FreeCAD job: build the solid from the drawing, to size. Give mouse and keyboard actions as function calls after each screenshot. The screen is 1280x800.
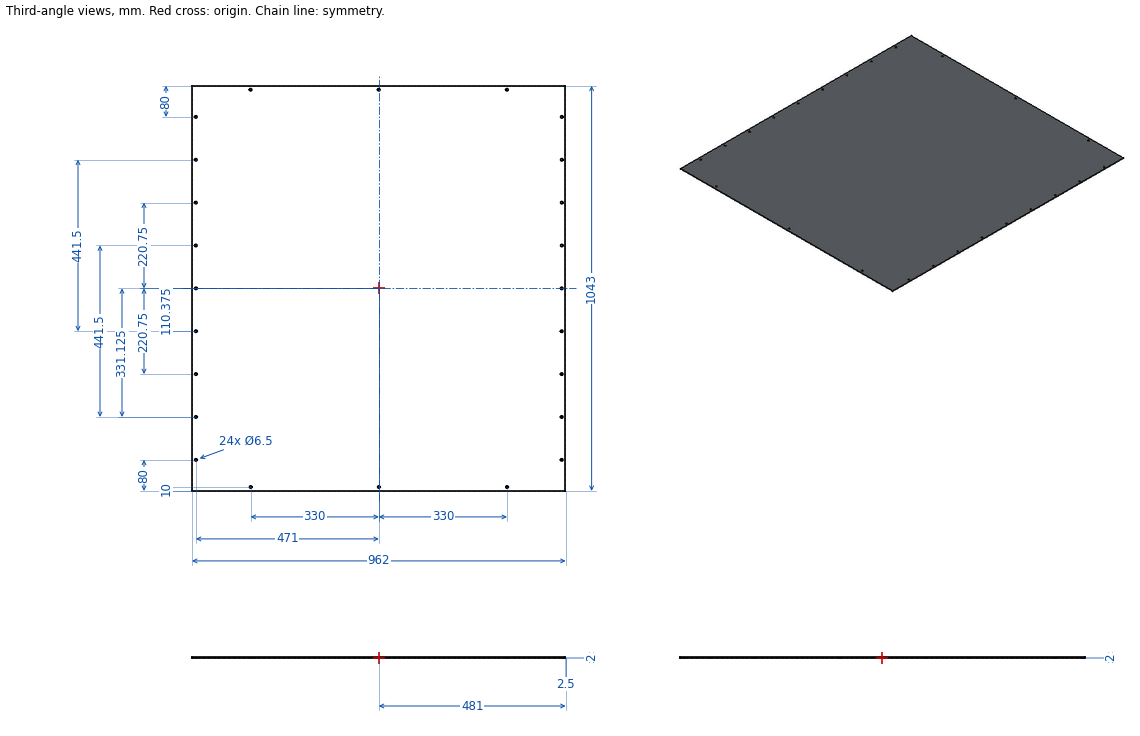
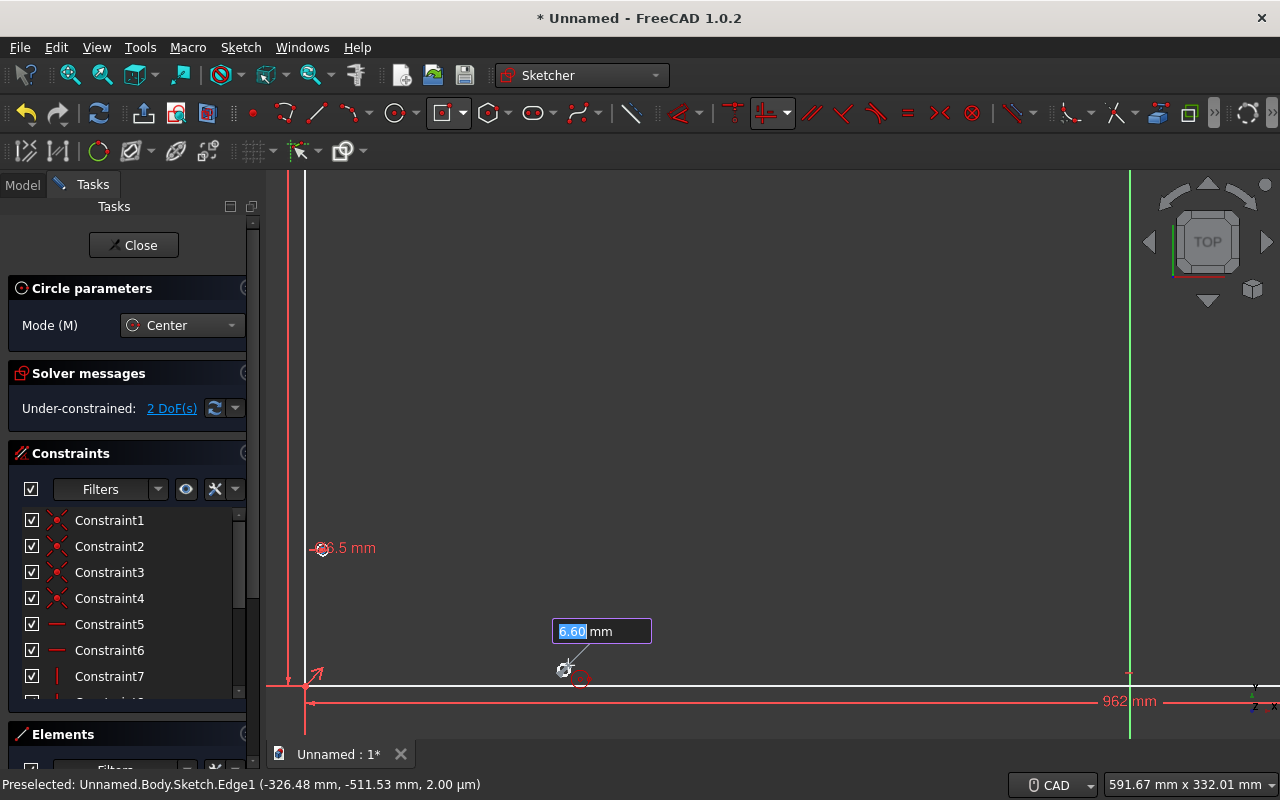
text(6.5)
key(Return)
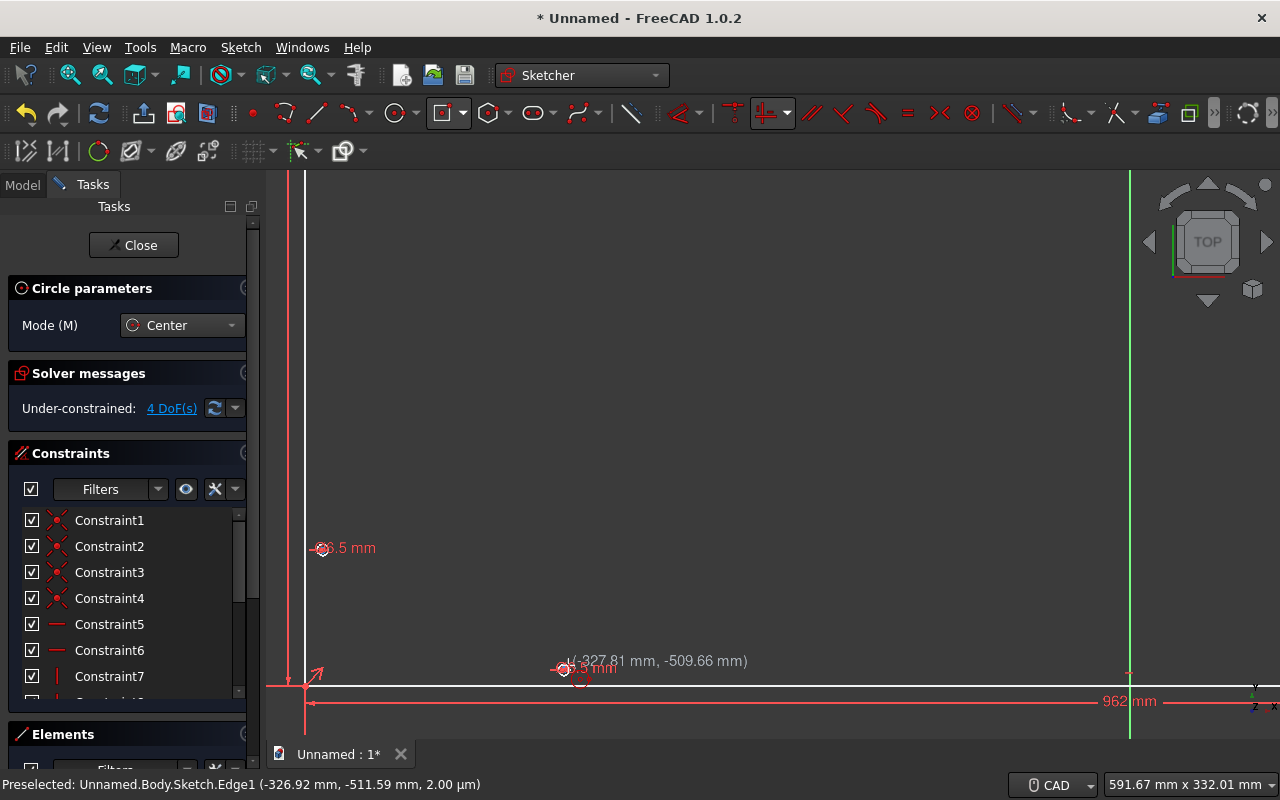
scroll(323, 360, up, 8)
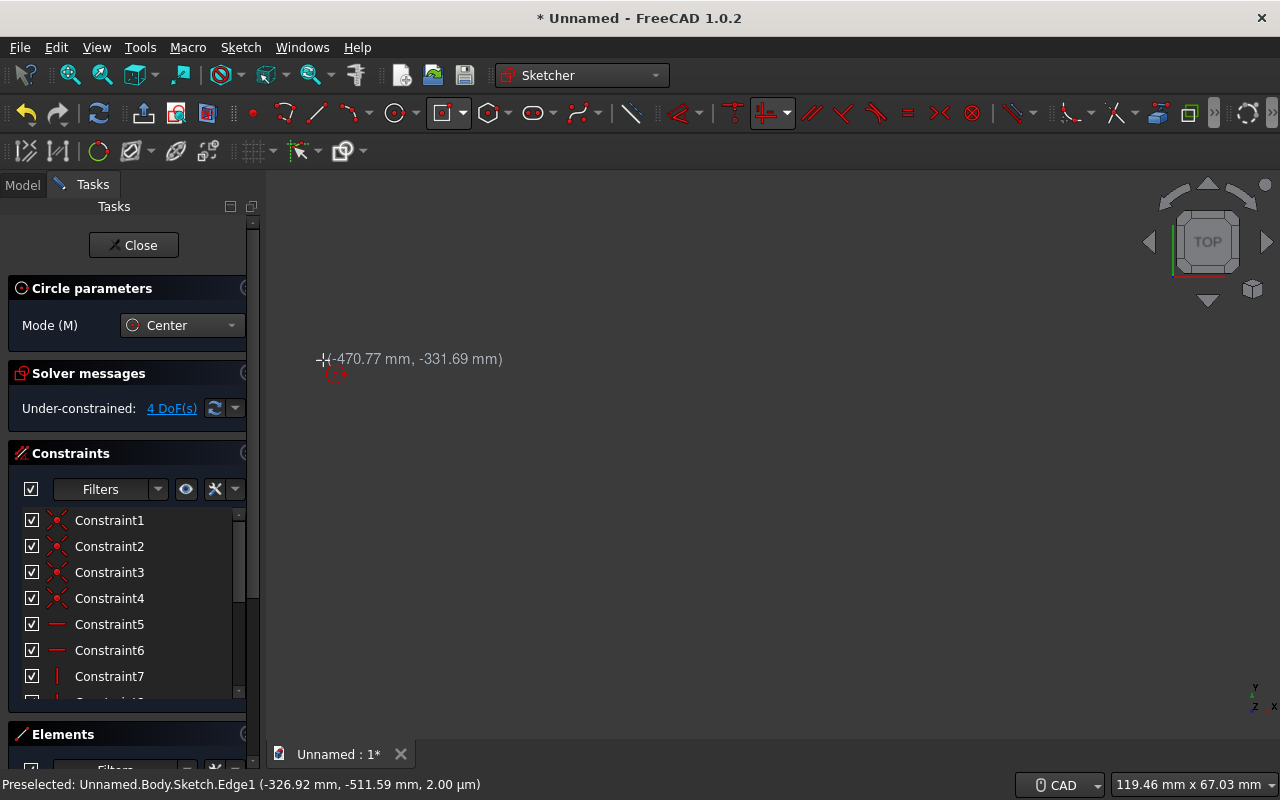
scroll(515, 607, down, 15)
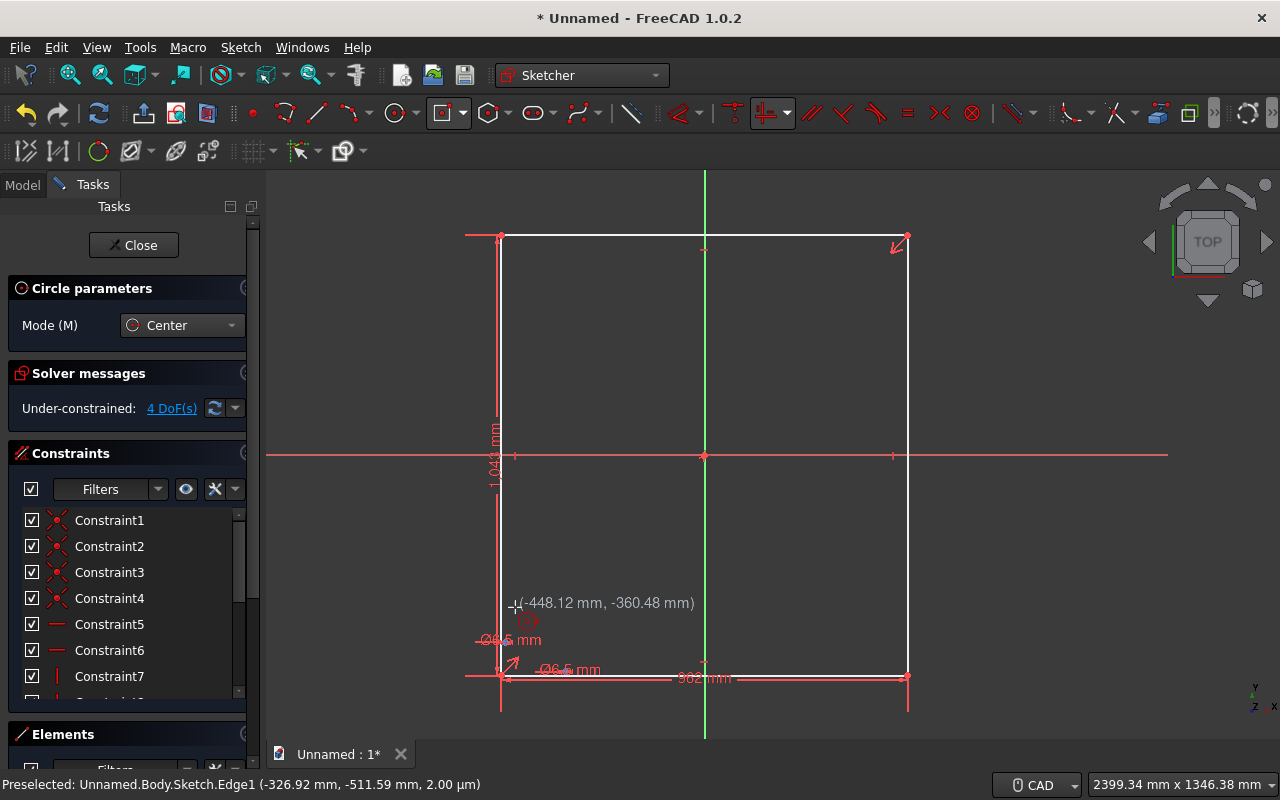
scroll(506, 595, up, 7)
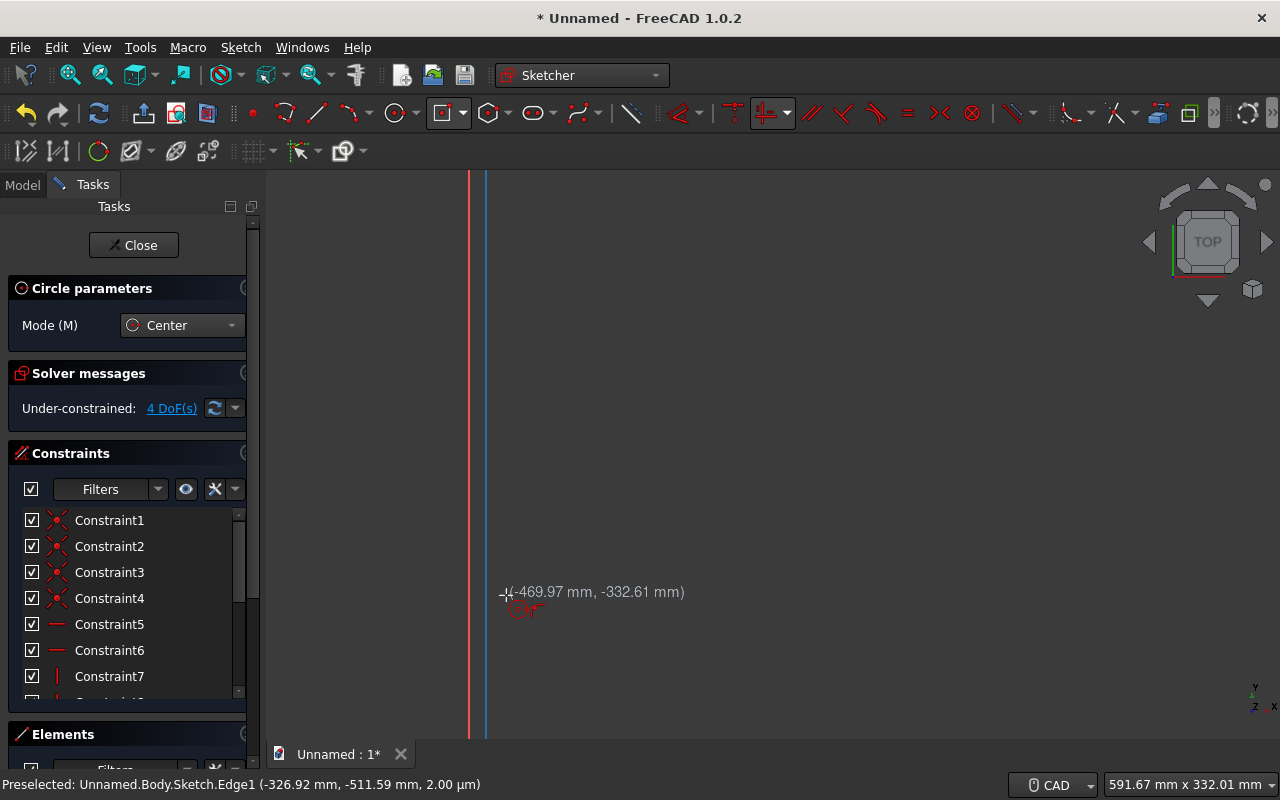
click(504, 594)
move(507, 590)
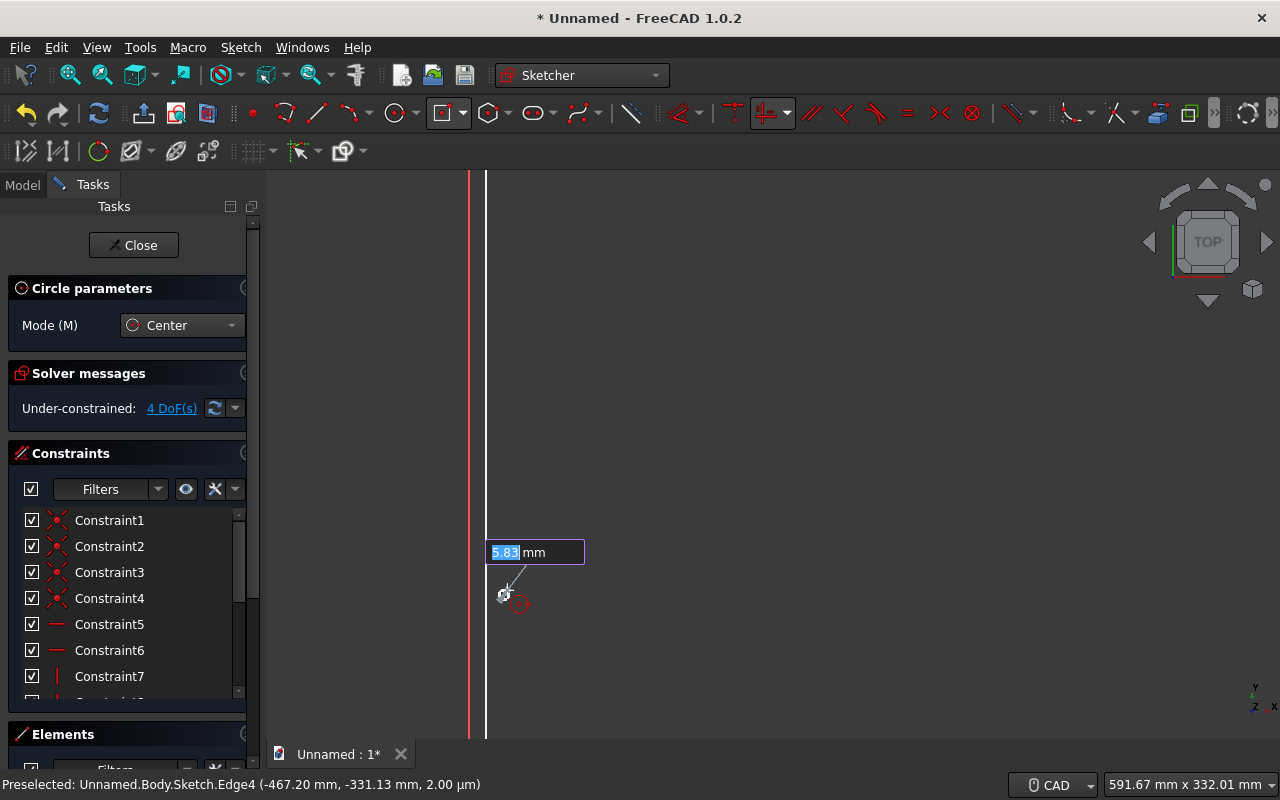
text(6.5)
key(Return)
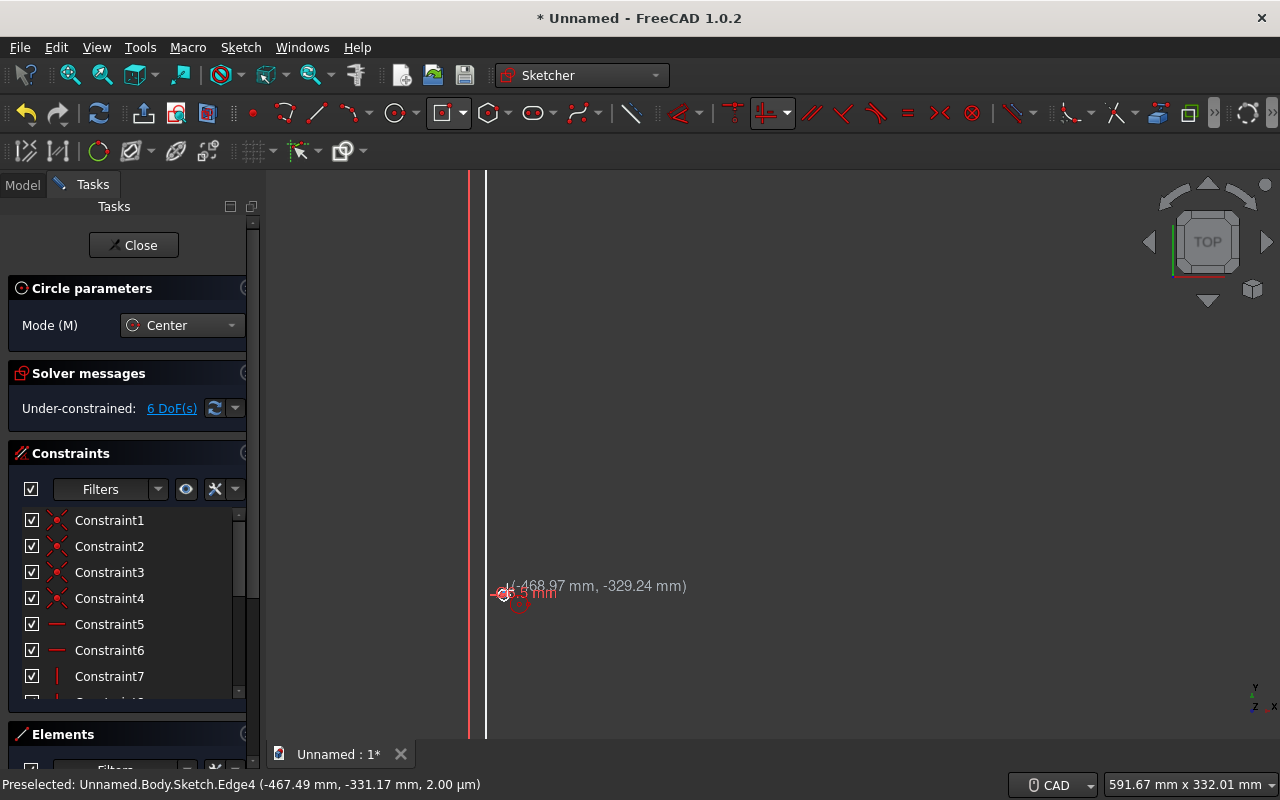
scroll(504, 405, up, 8)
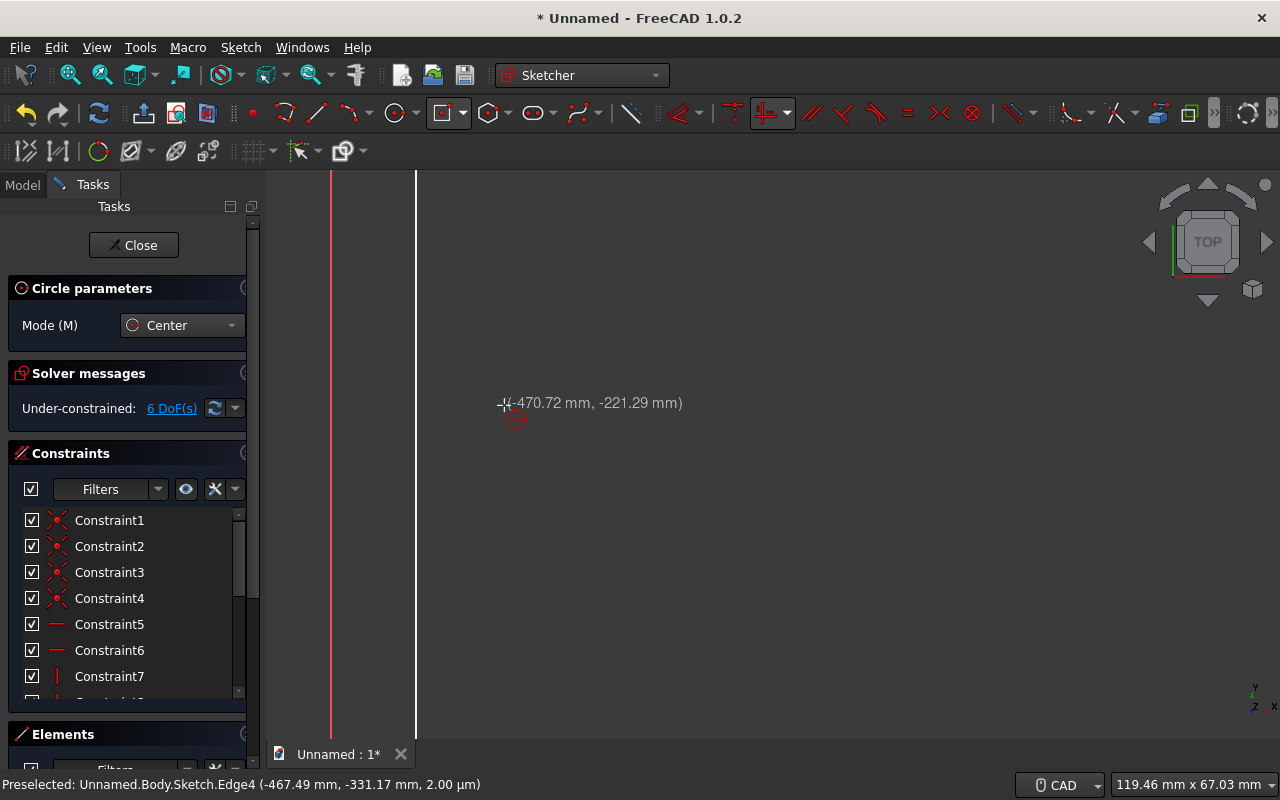
scroll(506, 555, down, 15)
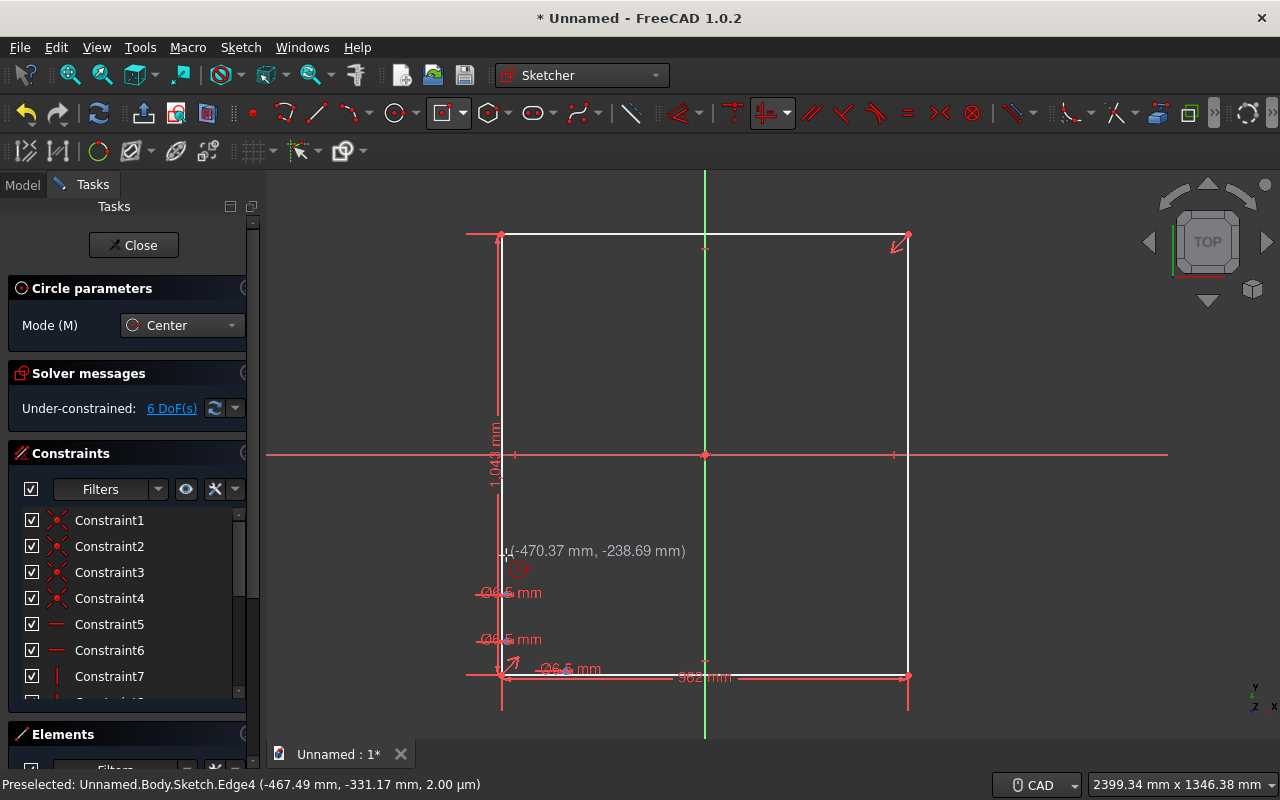
scroll(506, 548, up, 7)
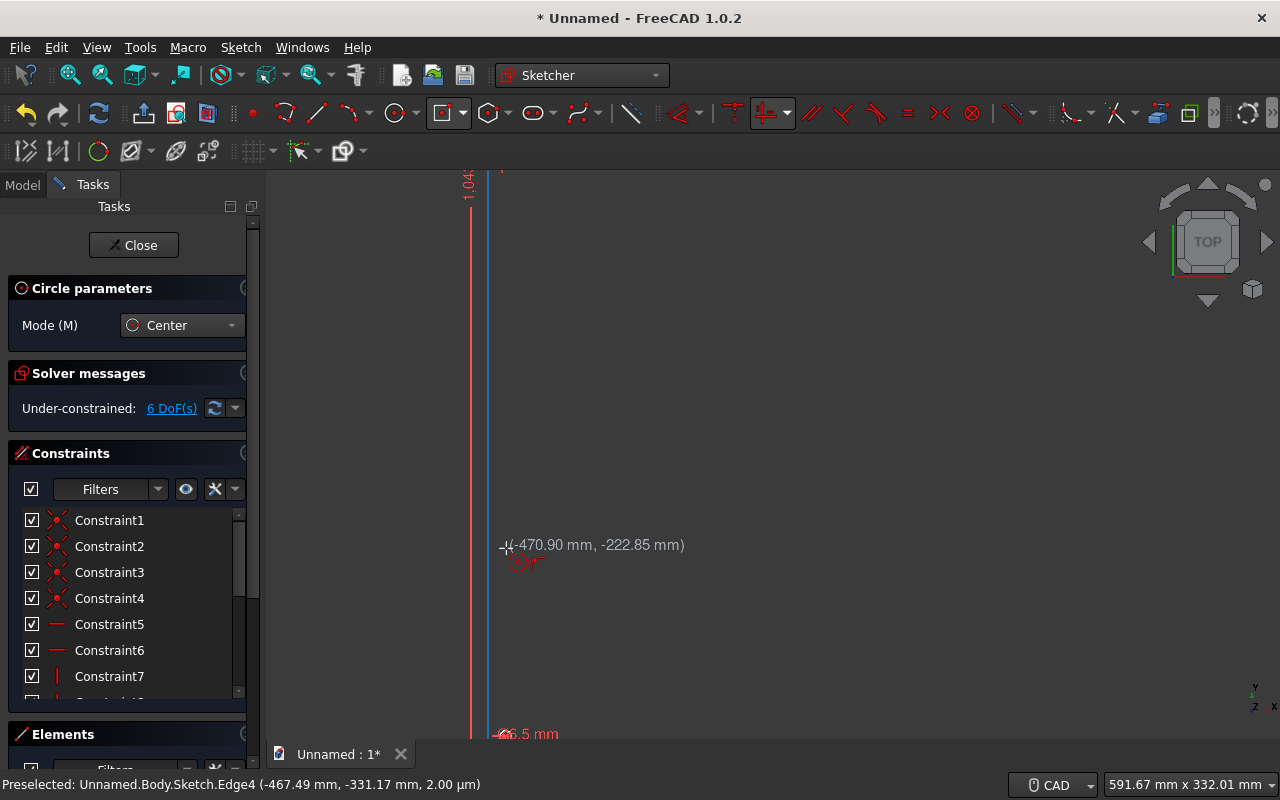
click(505, 546)
move(509, 542)